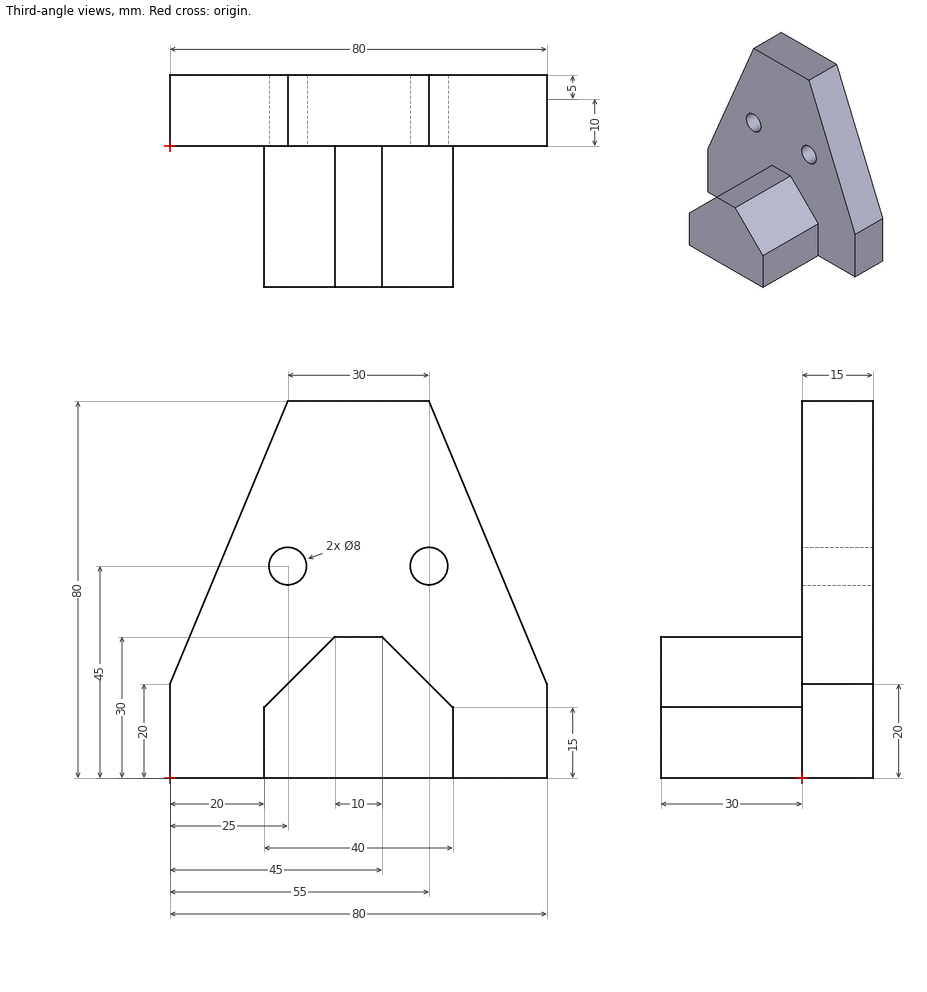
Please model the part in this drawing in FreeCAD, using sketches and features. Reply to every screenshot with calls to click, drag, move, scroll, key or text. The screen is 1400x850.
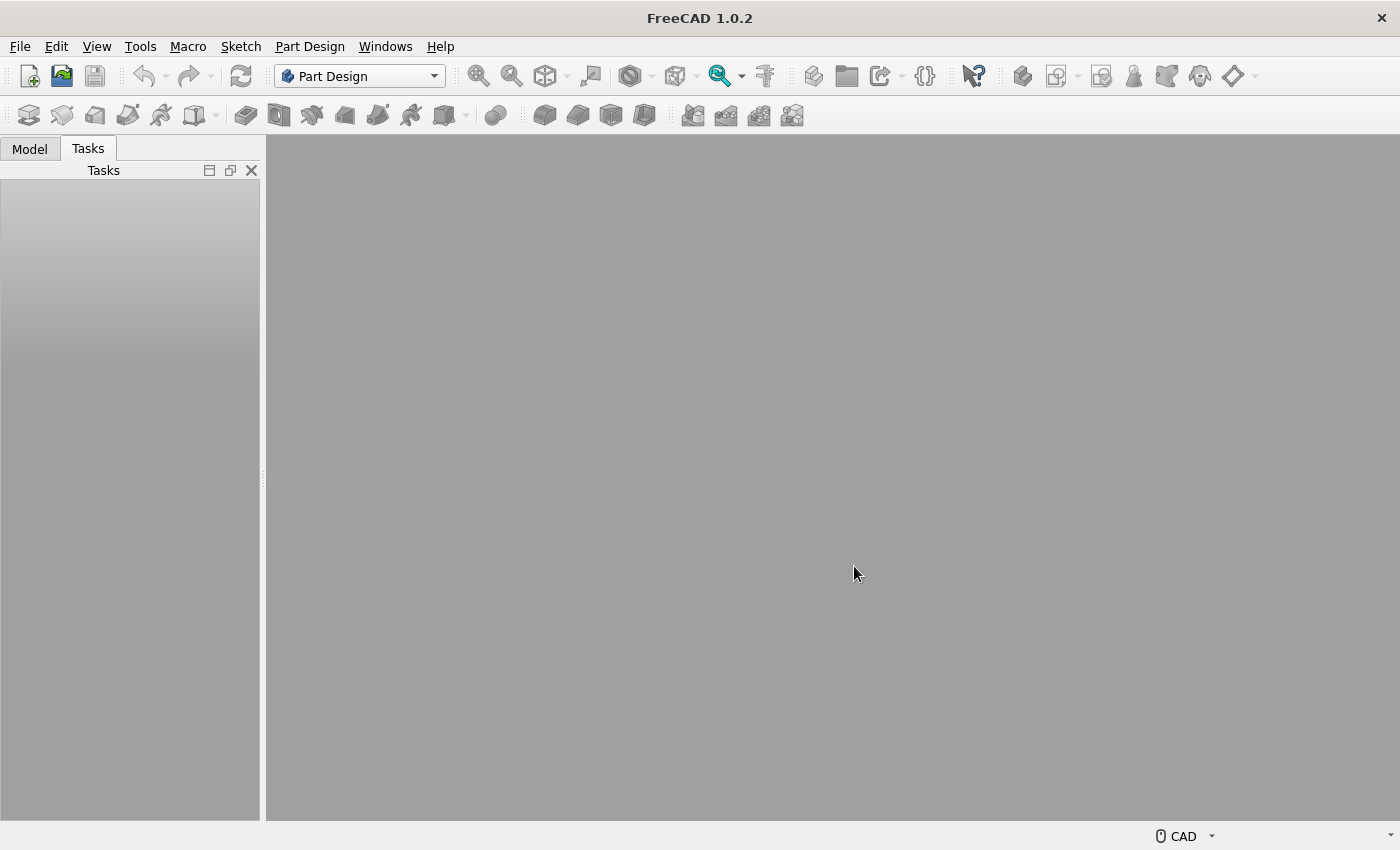
click(29, 76)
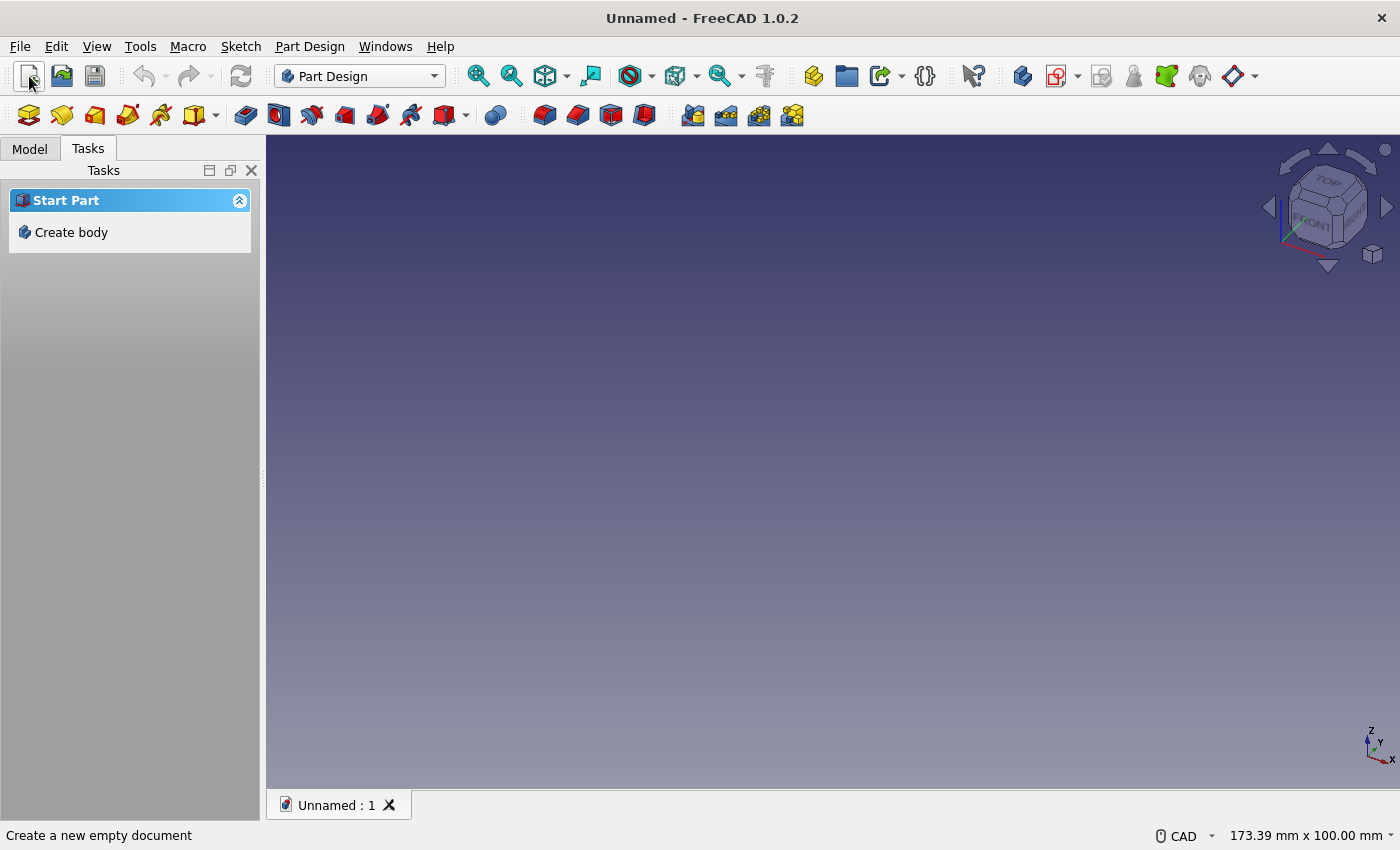
click(1056, 76)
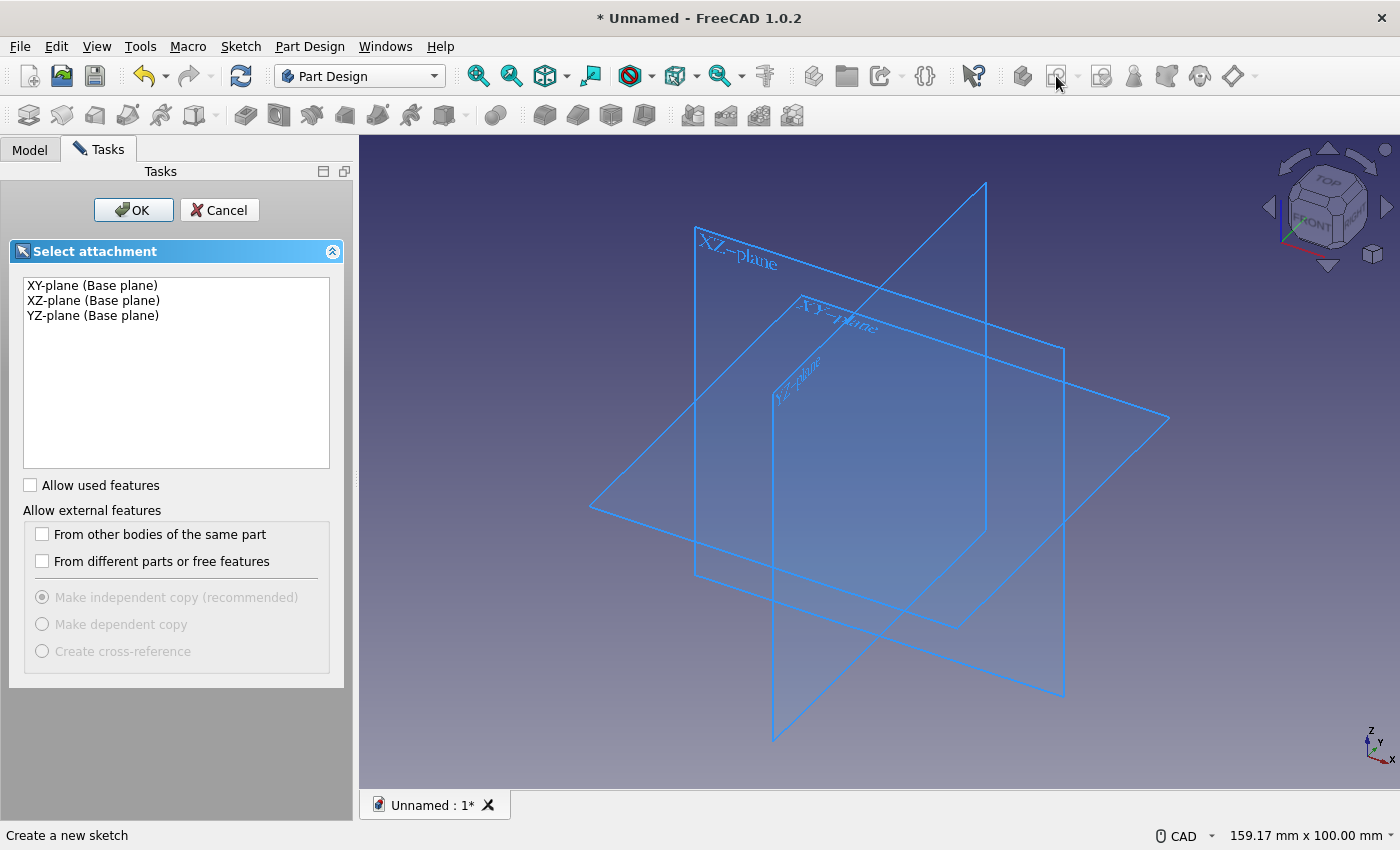
click(84, 286)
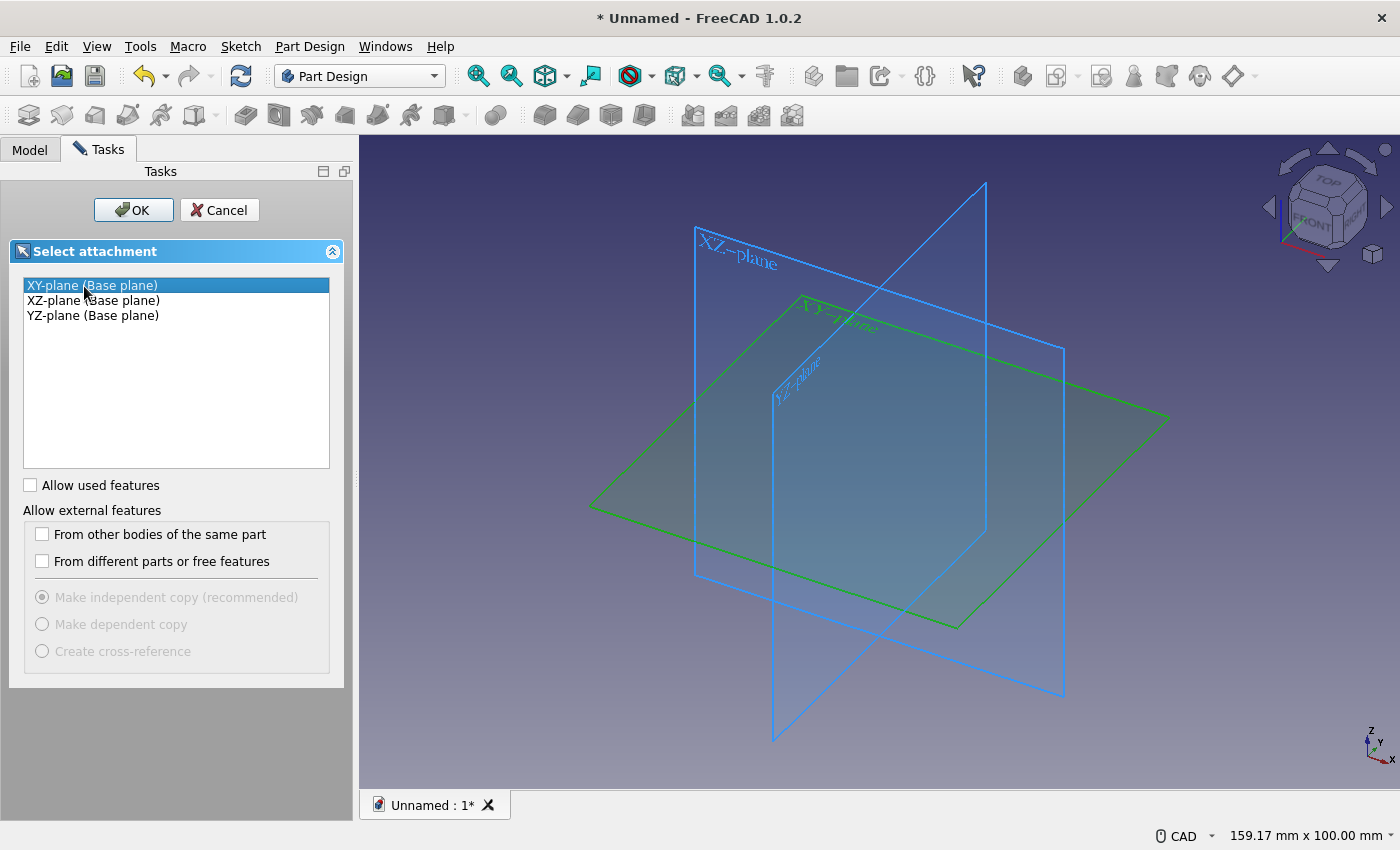
click(134, 210)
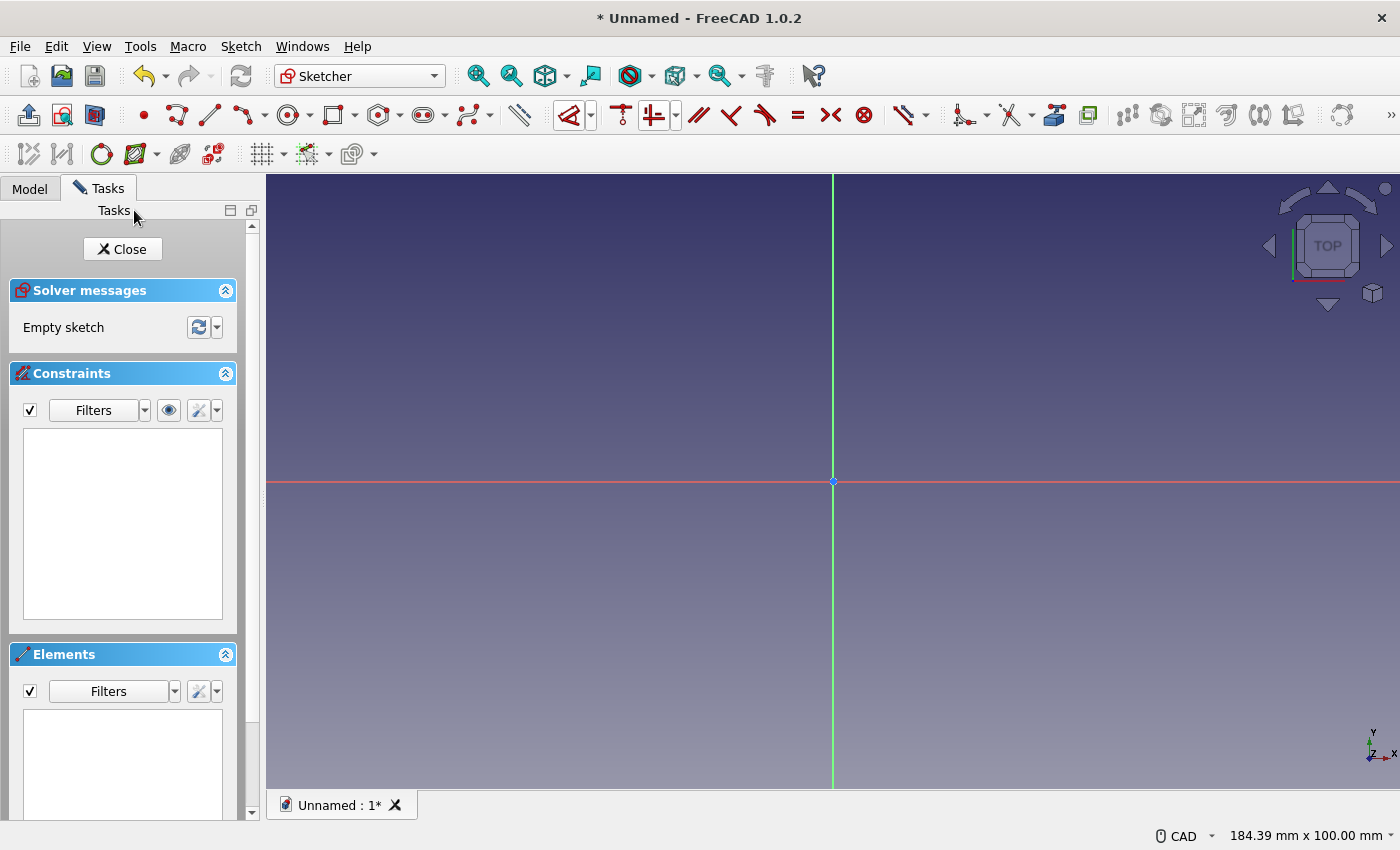
scroll(294, 620, down, 1)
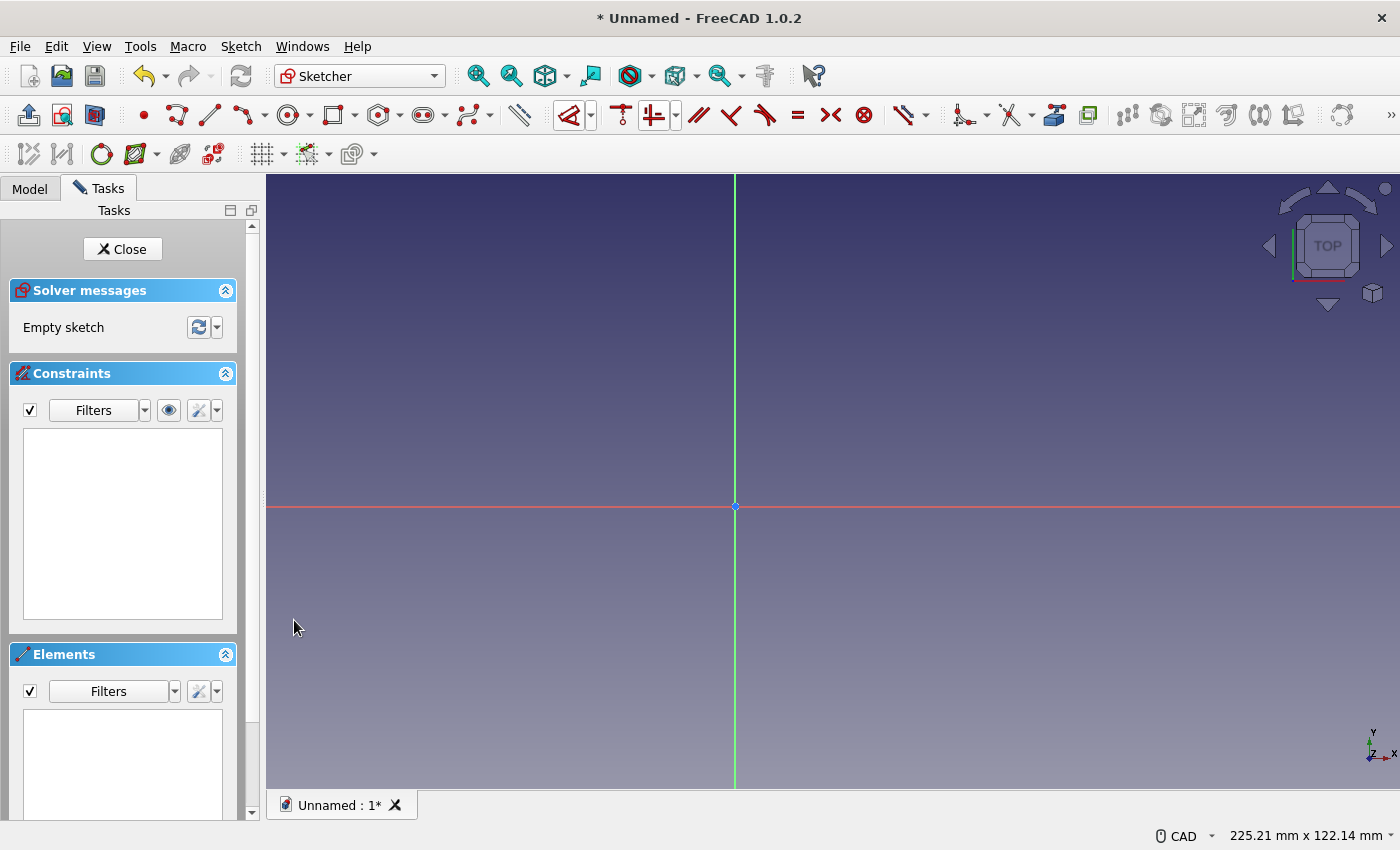
scroll(1146, 482, up, 3)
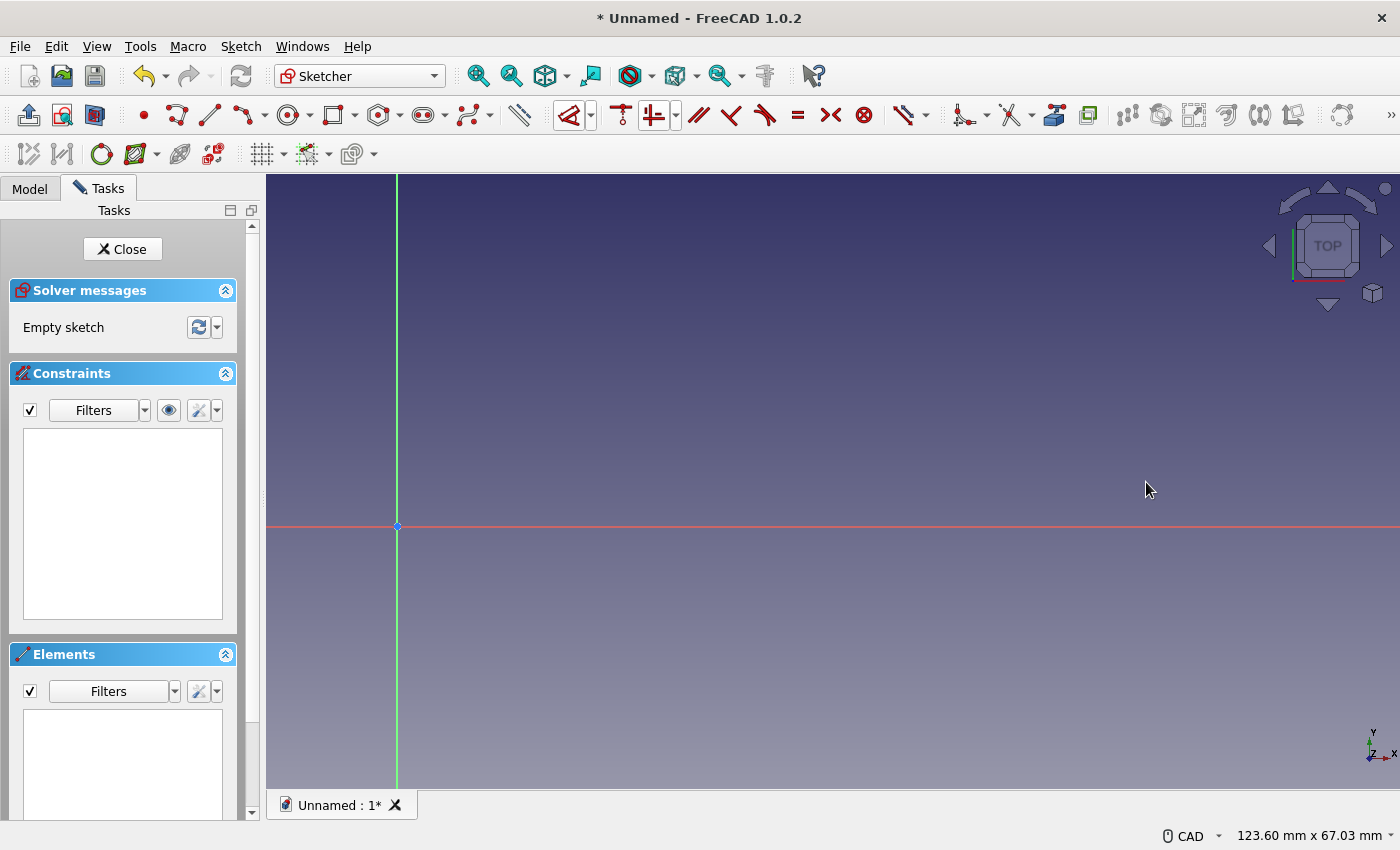
click(332, 116)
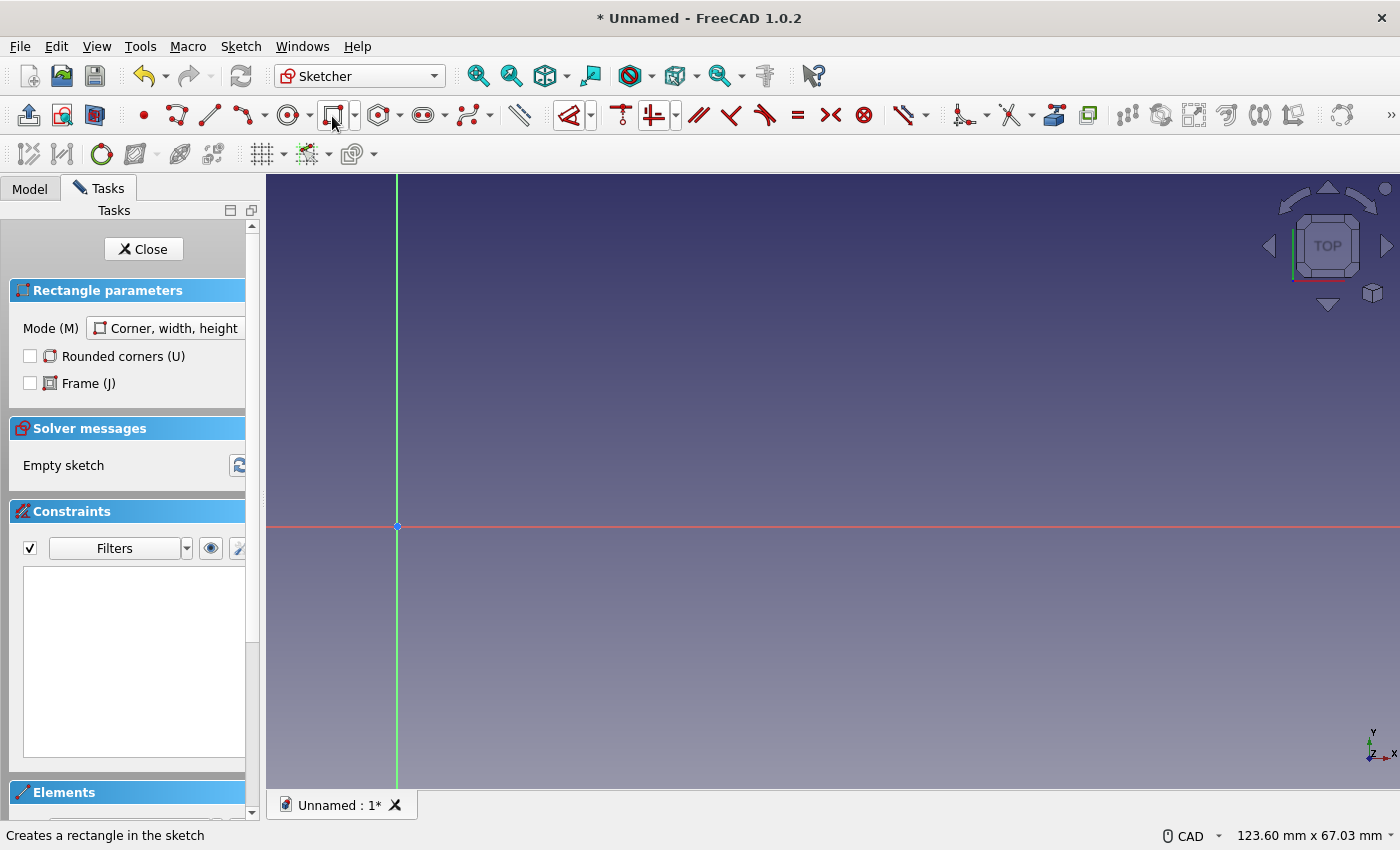
click(397, 527)
move(1131, 435)